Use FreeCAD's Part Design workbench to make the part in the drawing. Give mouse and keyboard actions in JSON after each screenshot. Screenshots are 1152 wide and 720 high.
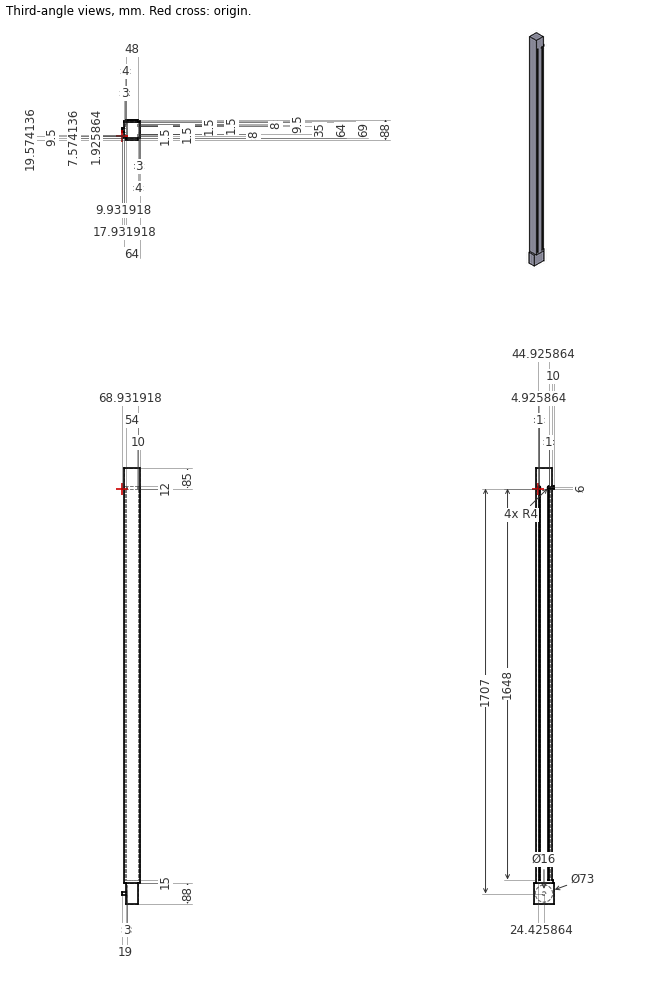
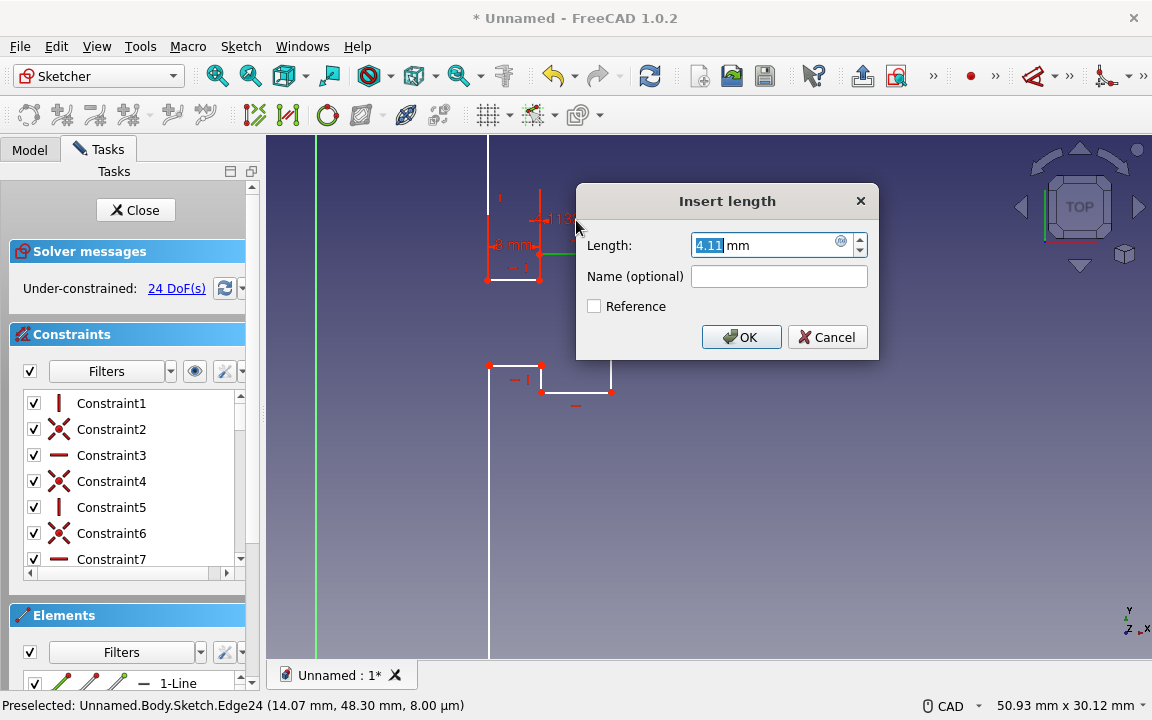
{"action": "type", "text": "4"}
{"action": "key", "text": "Return"}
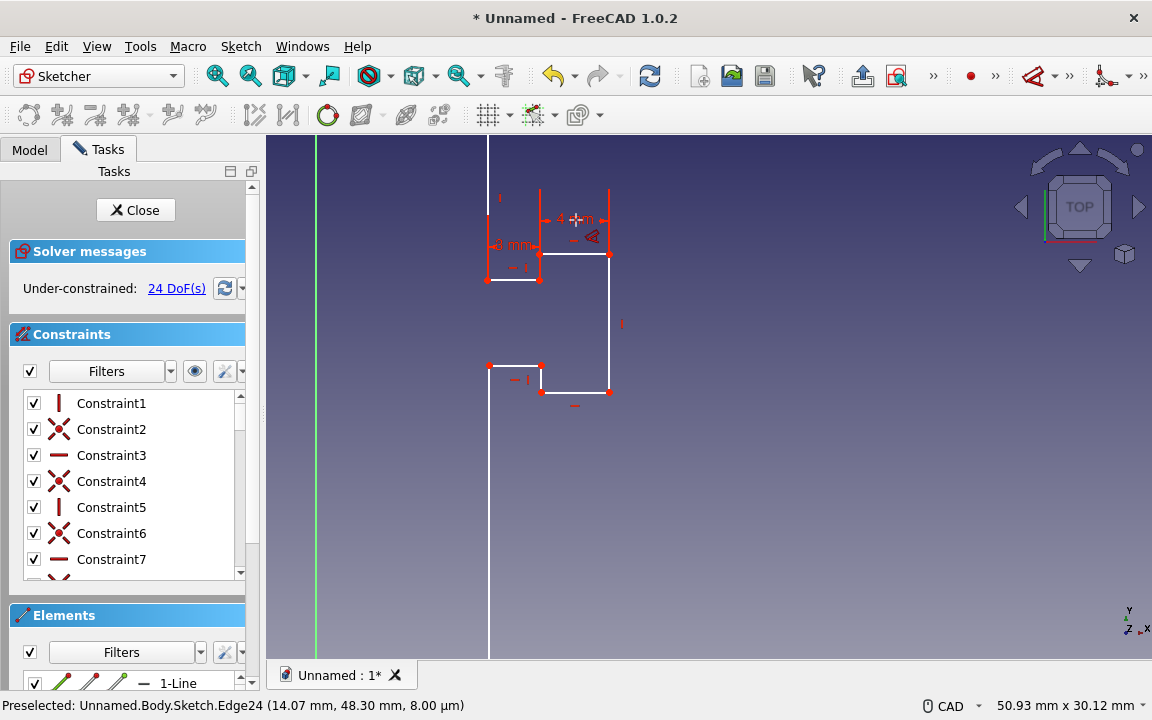
{"action": "scroll", "coordinate": [503, 280], "scroll_direction": "down", "scroll_amount": 6}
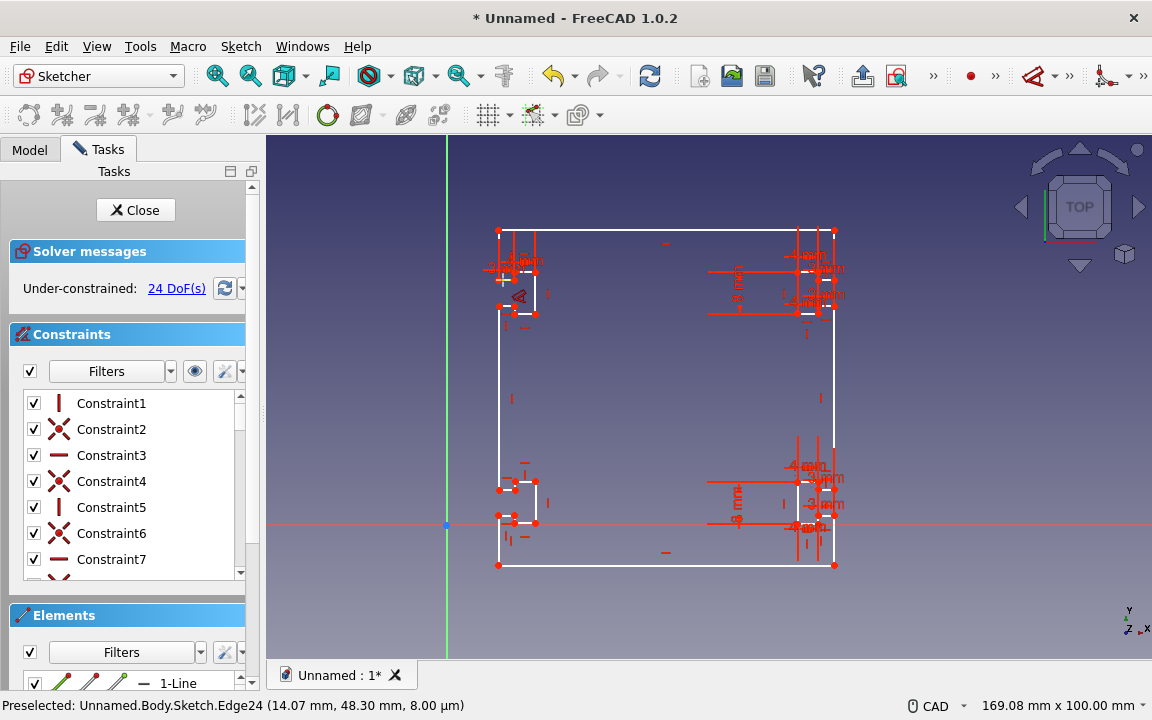
{"action": "left_click", "coordinate": [535, 285]}
{"action": "left_click", "coordinate": [569, 293]}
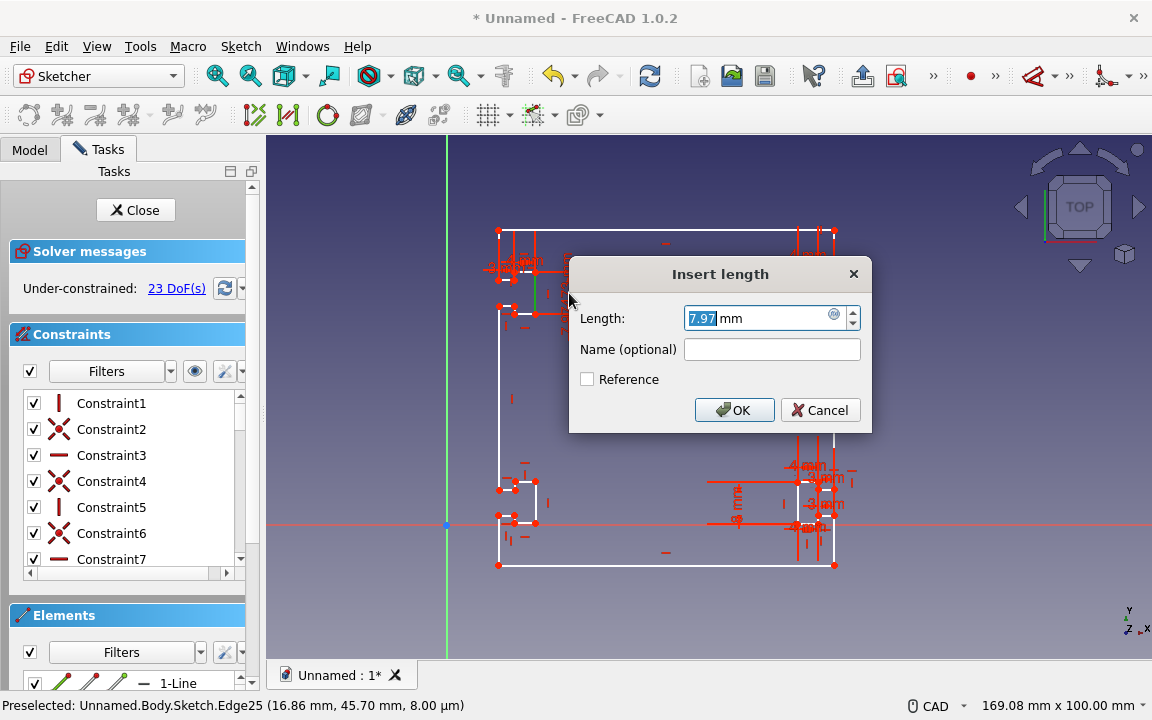
{"action": "type", "text": "8"}
{"action": "key", "text": "Return"}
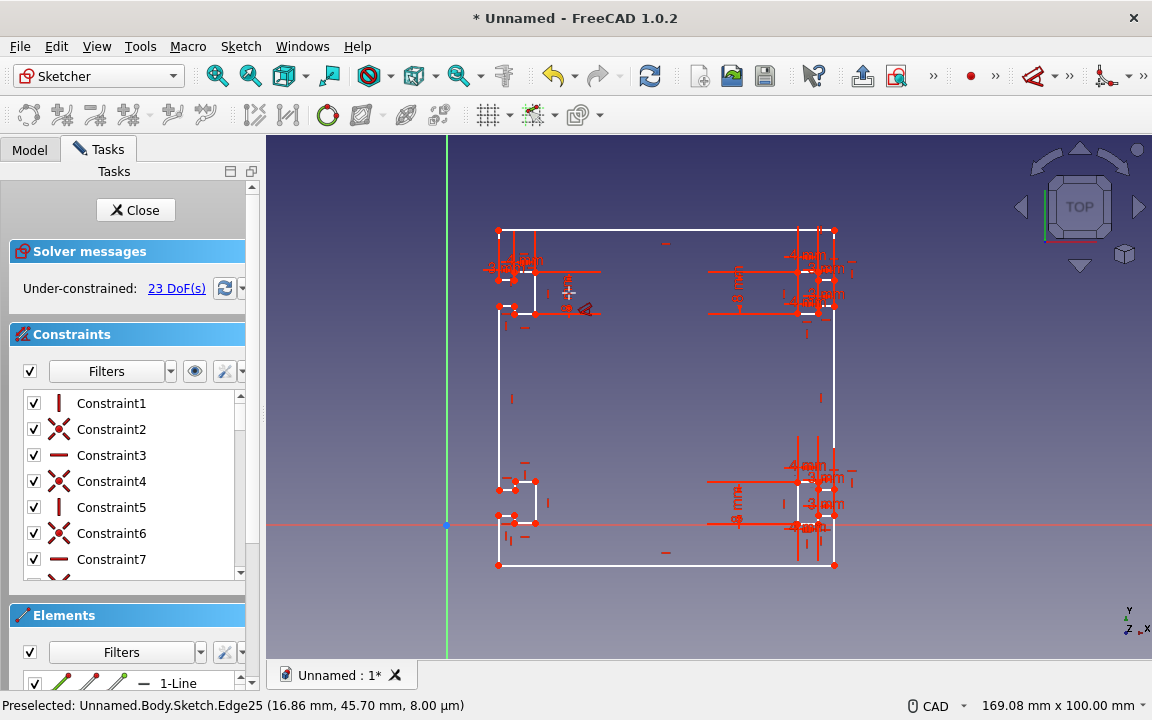
{"action": "scroll", "coordinate": [525, 314], "scroll_direction": "up", "scroll_amount": 4}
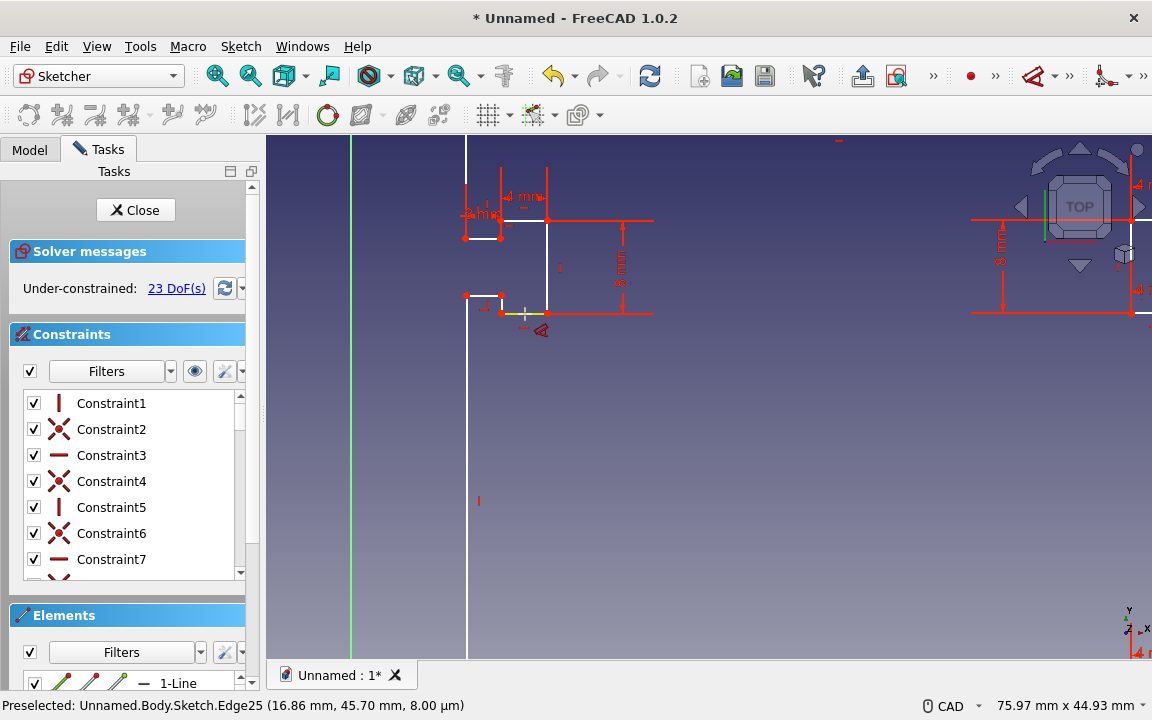
{"action": "left_click", "coordinate": [525, 314]}
{"action": "left_click", "coordinate": [525, 280]}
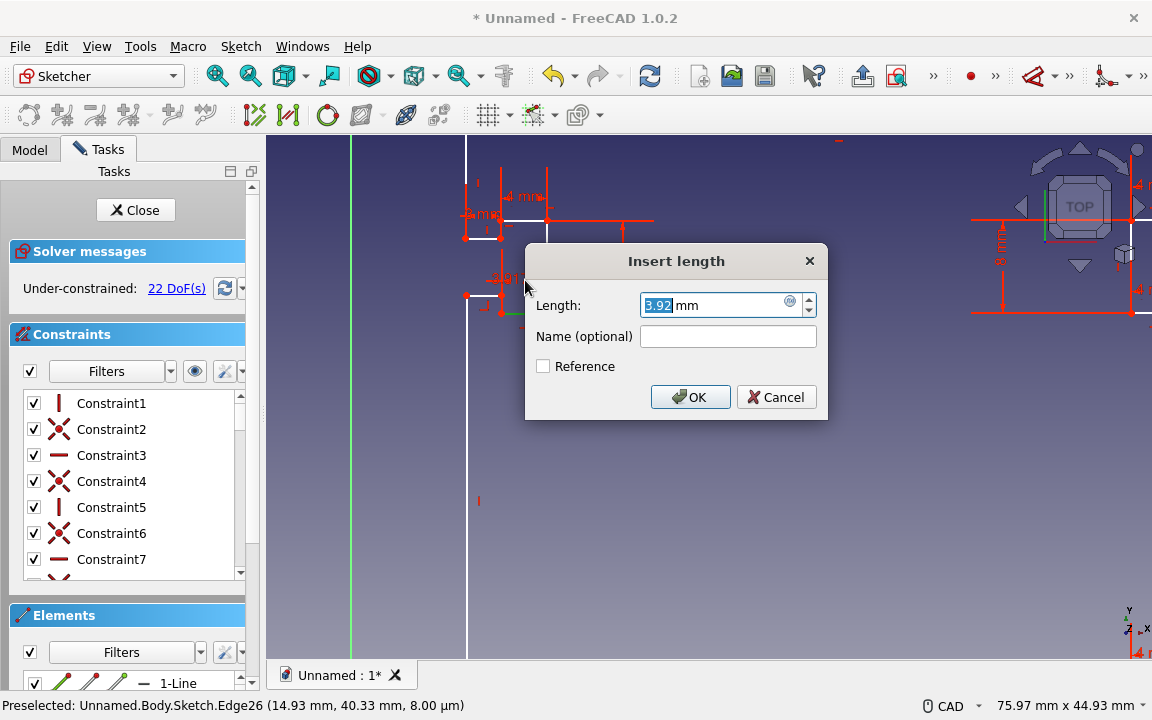
{"action": "type", "text": "4"}
{"action": "key", "text": "Return"}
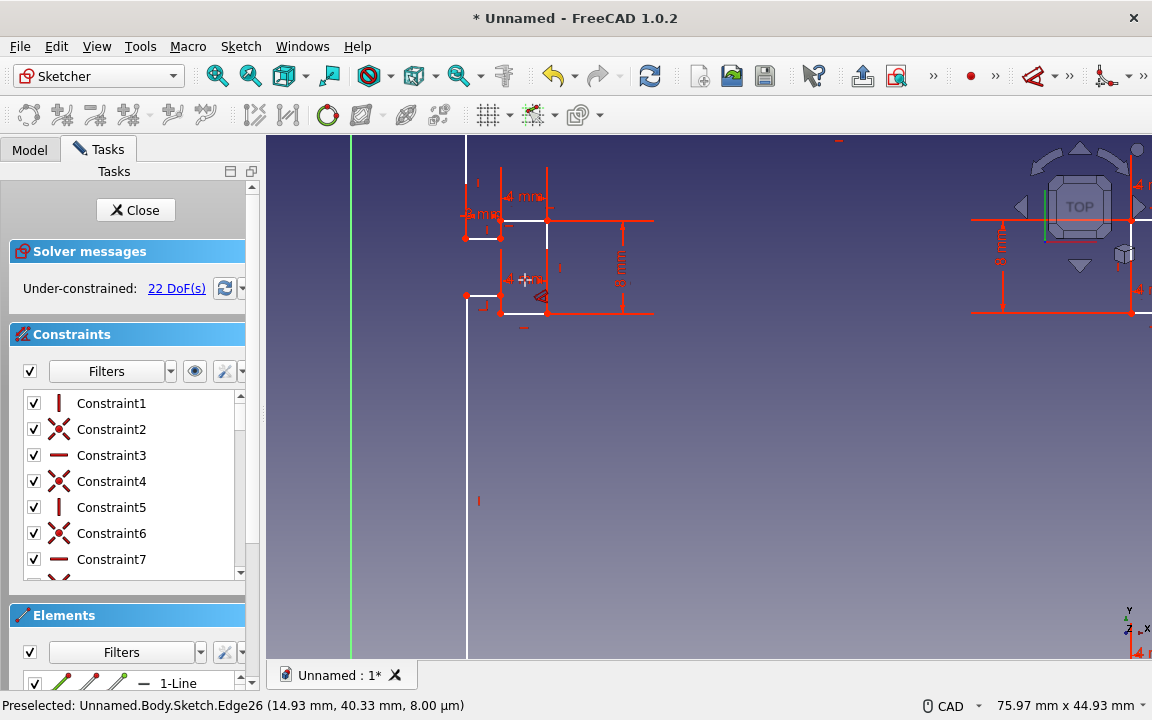
{"action": "scroll", "coordinate": [491, 296], "scroll_direction": "up", "scroll_amount": 2}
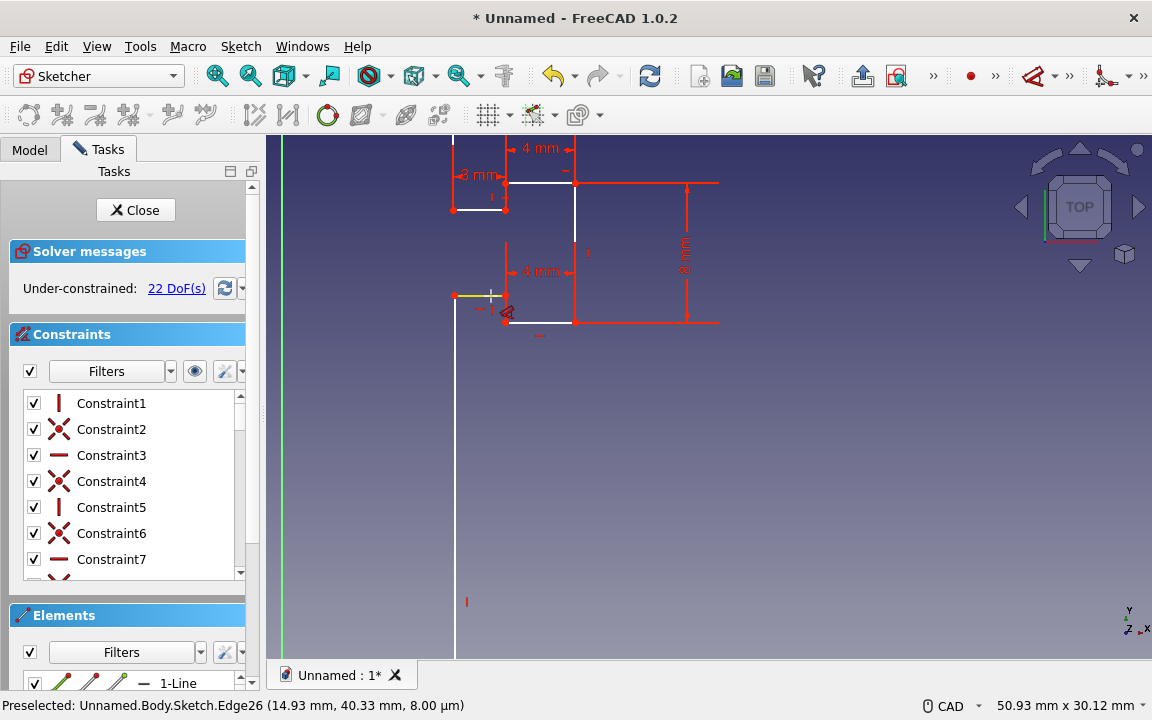
{"action": "left_click", "coordinate": [490, 296]}
{"action": "left_click", "coordinate": [468, 262]}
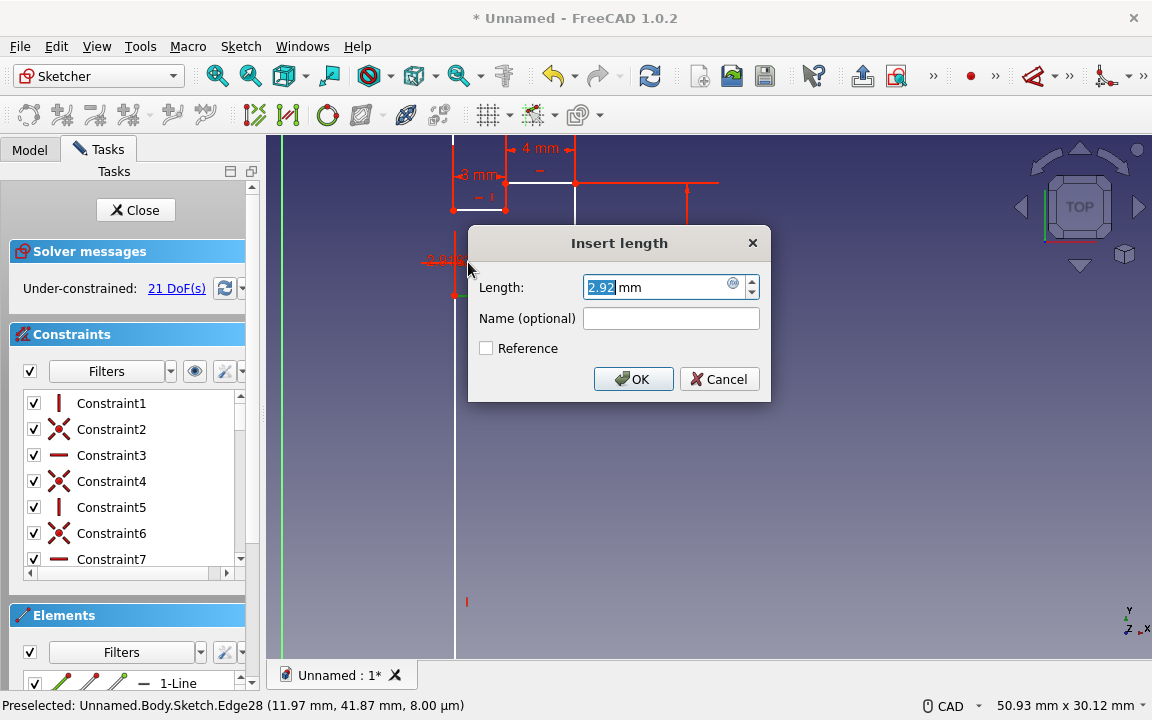
{"action": "type", "text": "3"}
{"action": "key", "text": "Return"}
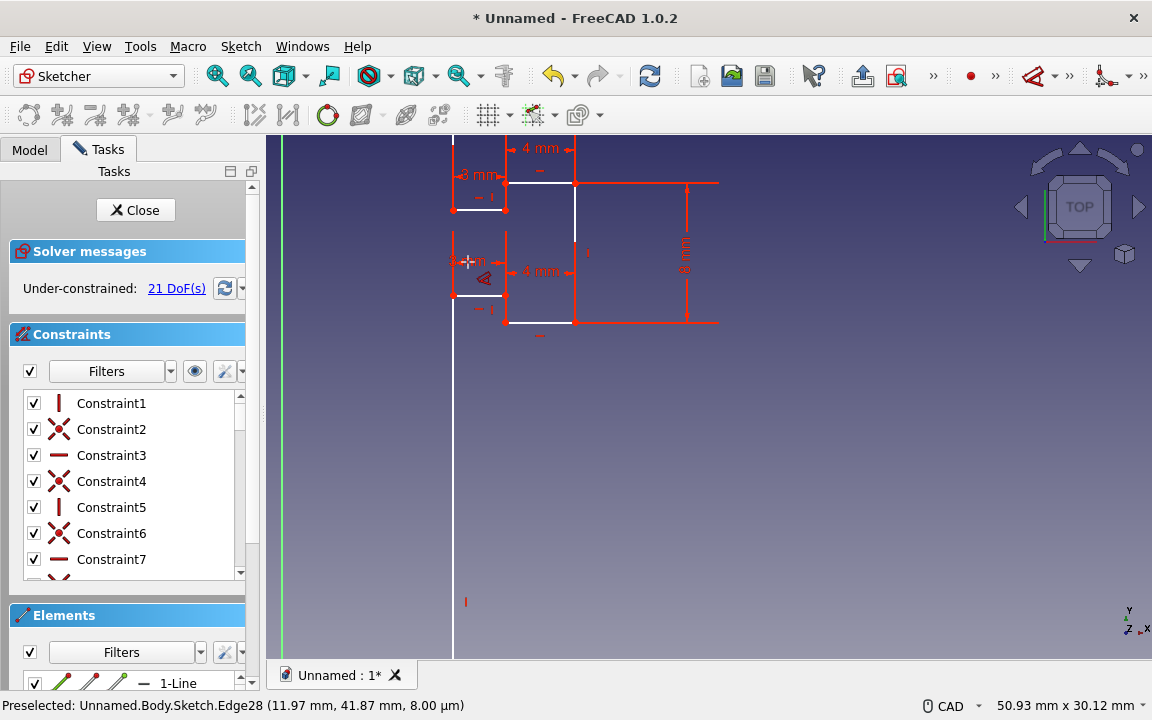
{"action": "scroll", "coordinate": [518, 310], "scroll_direction": "down", "scroll_amount": 6}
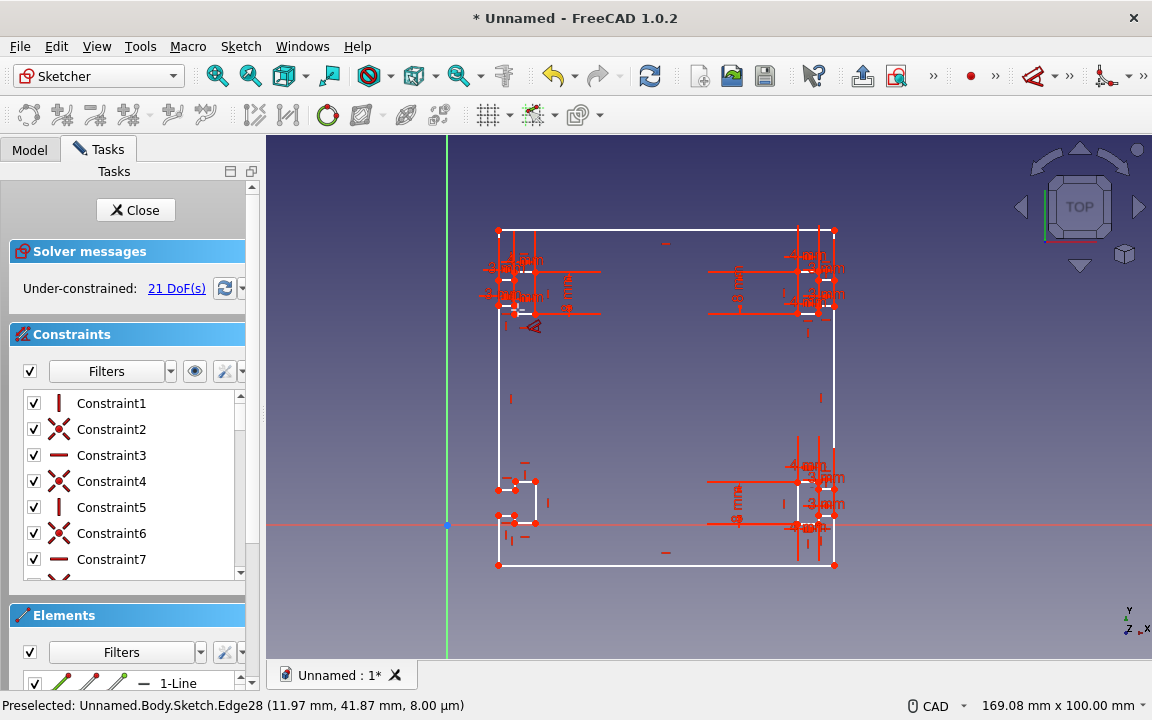
{"action": "scroll", "coordinate": [504, 490], "scroll_direction": "up", "scroll_amount": 6}